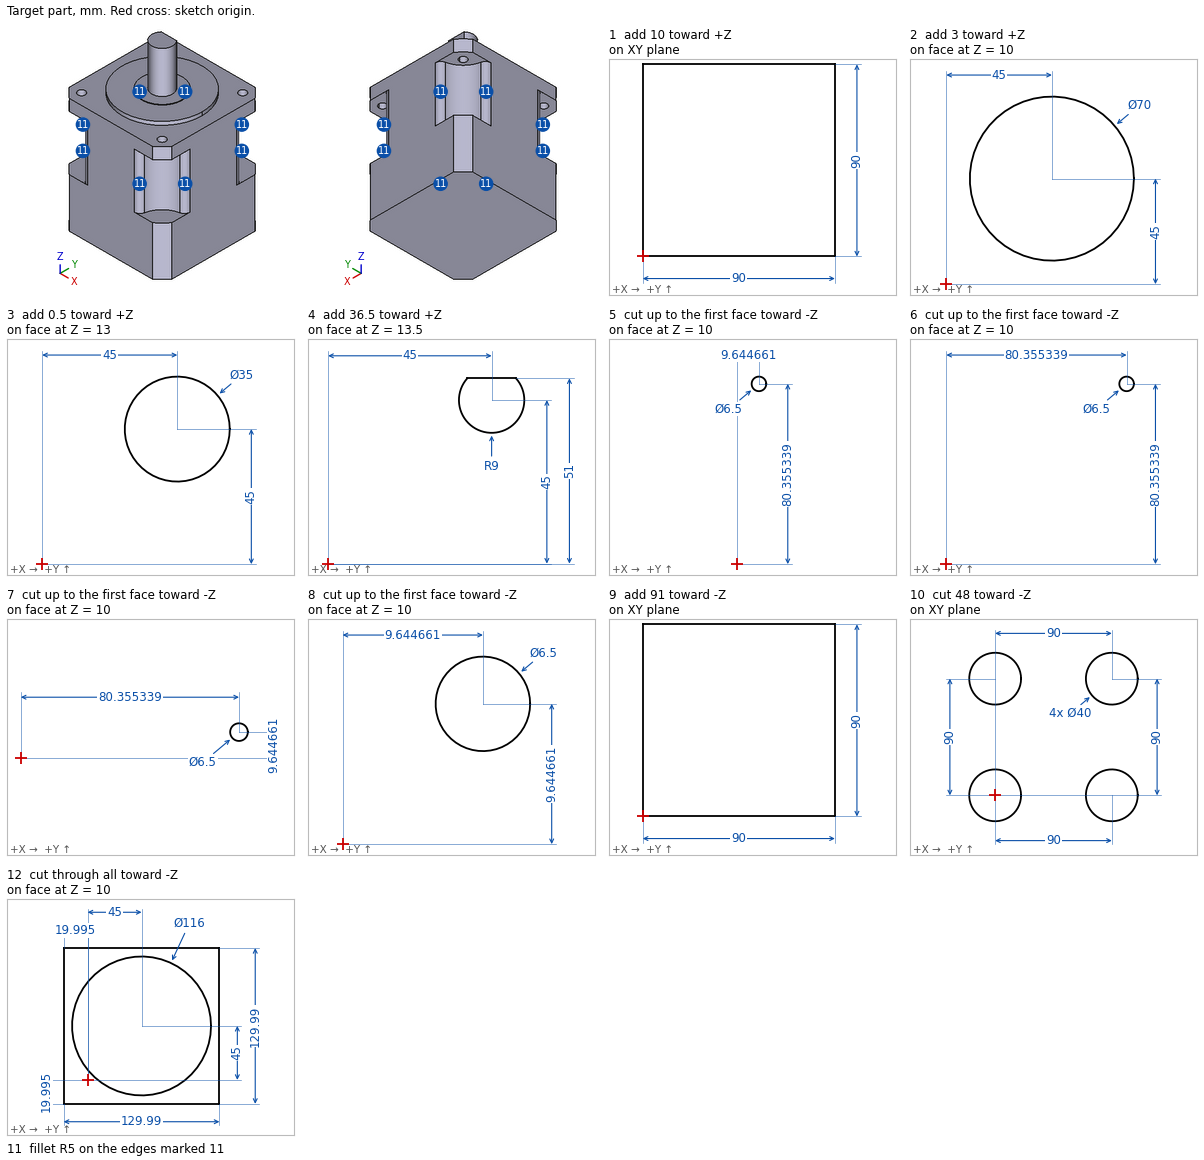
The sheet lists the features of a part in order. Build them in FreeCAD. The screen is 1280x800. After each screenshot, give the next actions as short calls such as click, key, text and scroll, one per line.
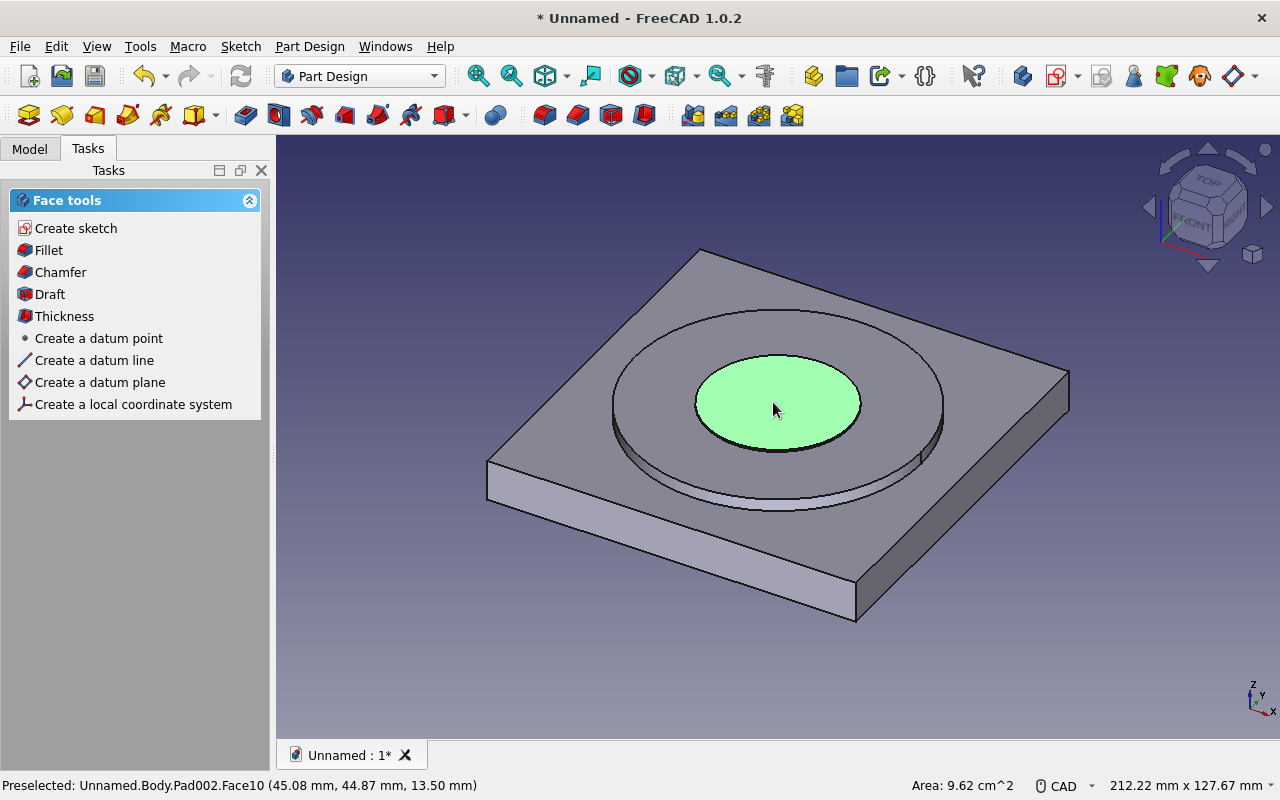
click(1056, 76)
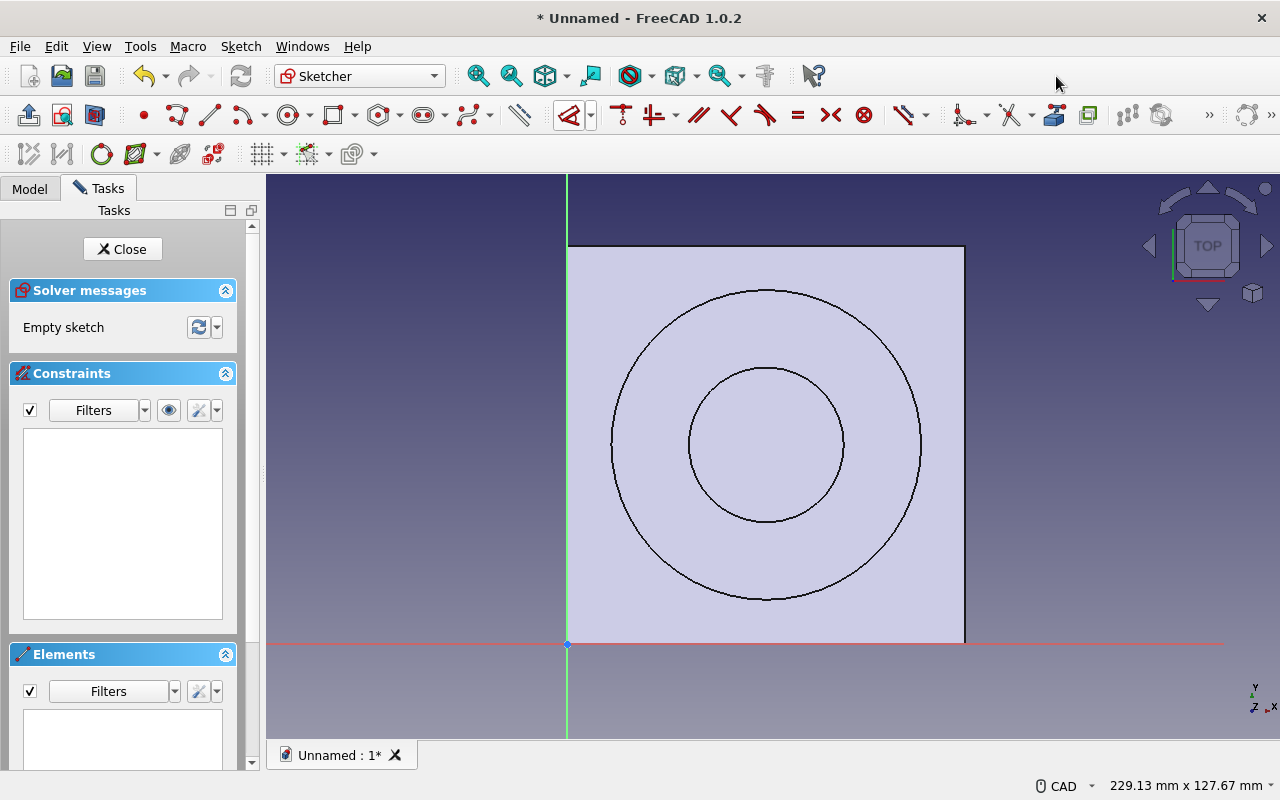
scroll(782, 450, up, 8)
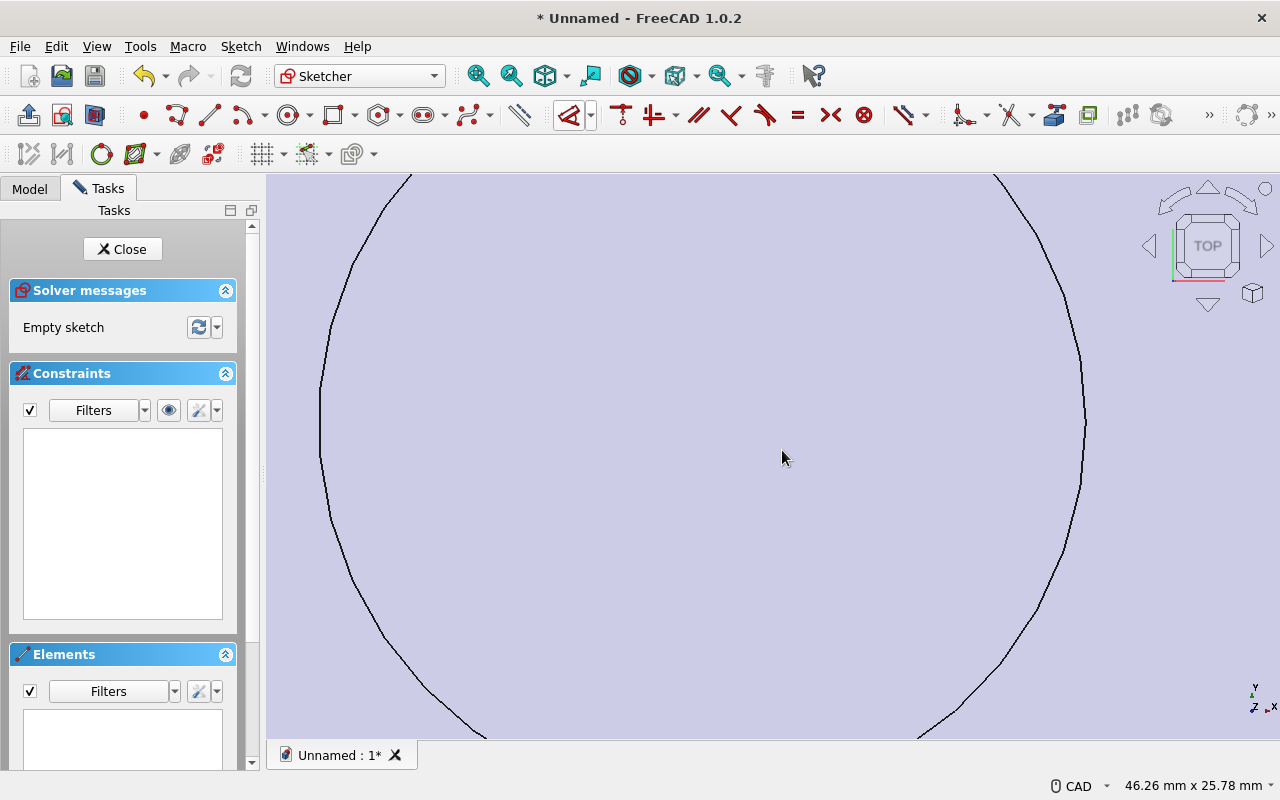
click(210, 116)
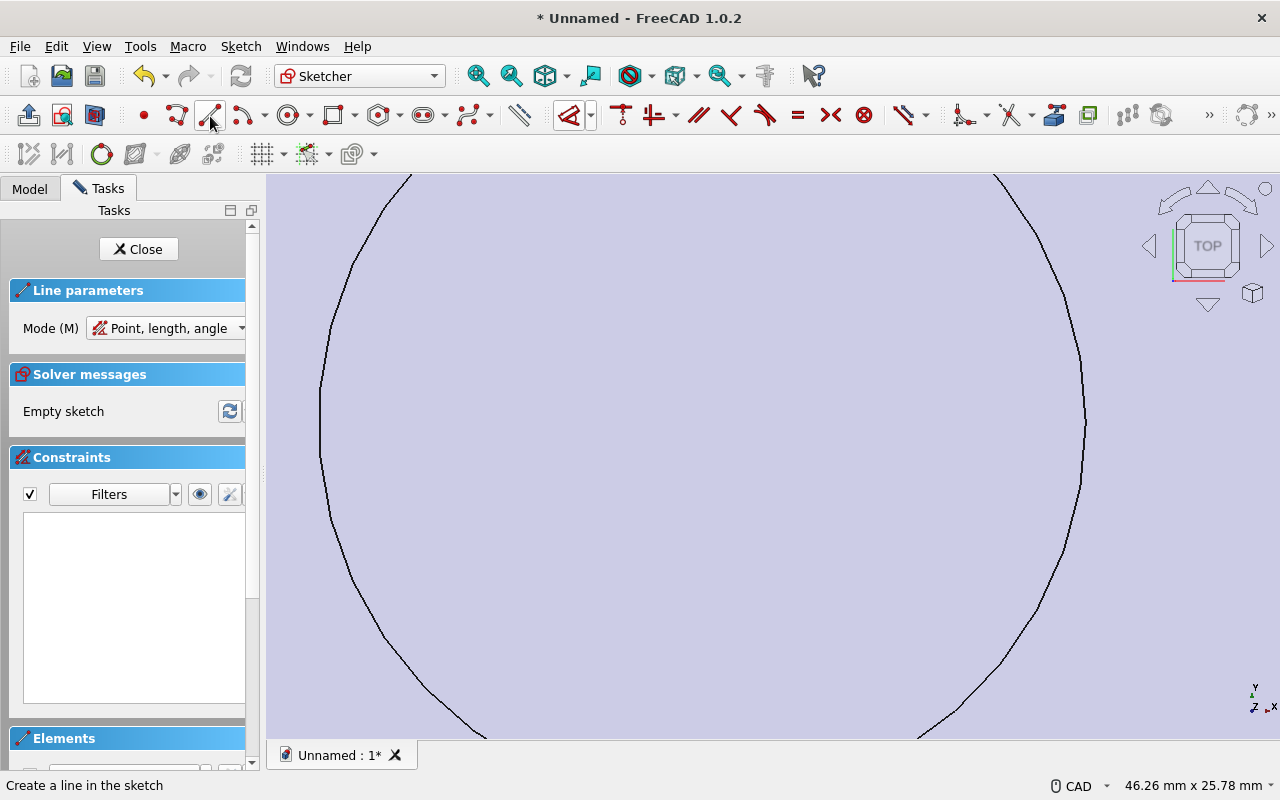
click(849, 291)
click(555, 291)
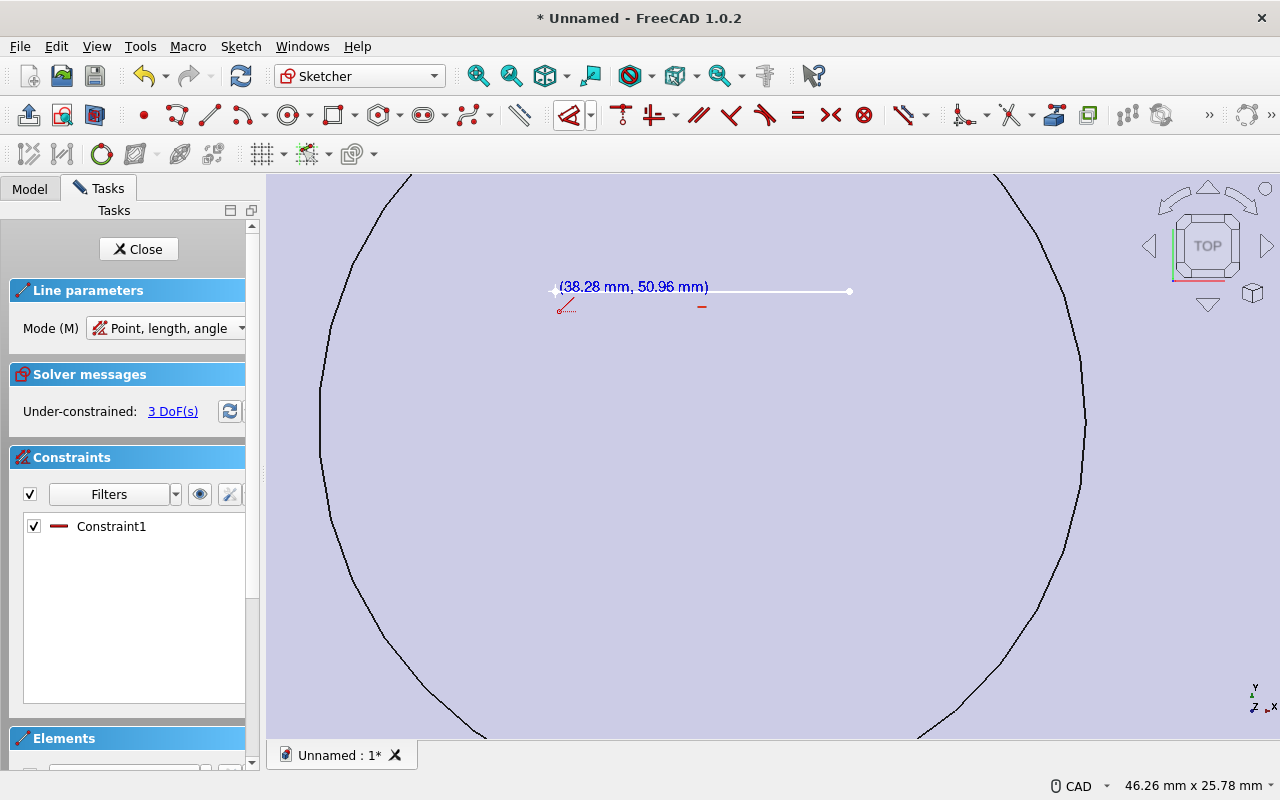
click(264, 116)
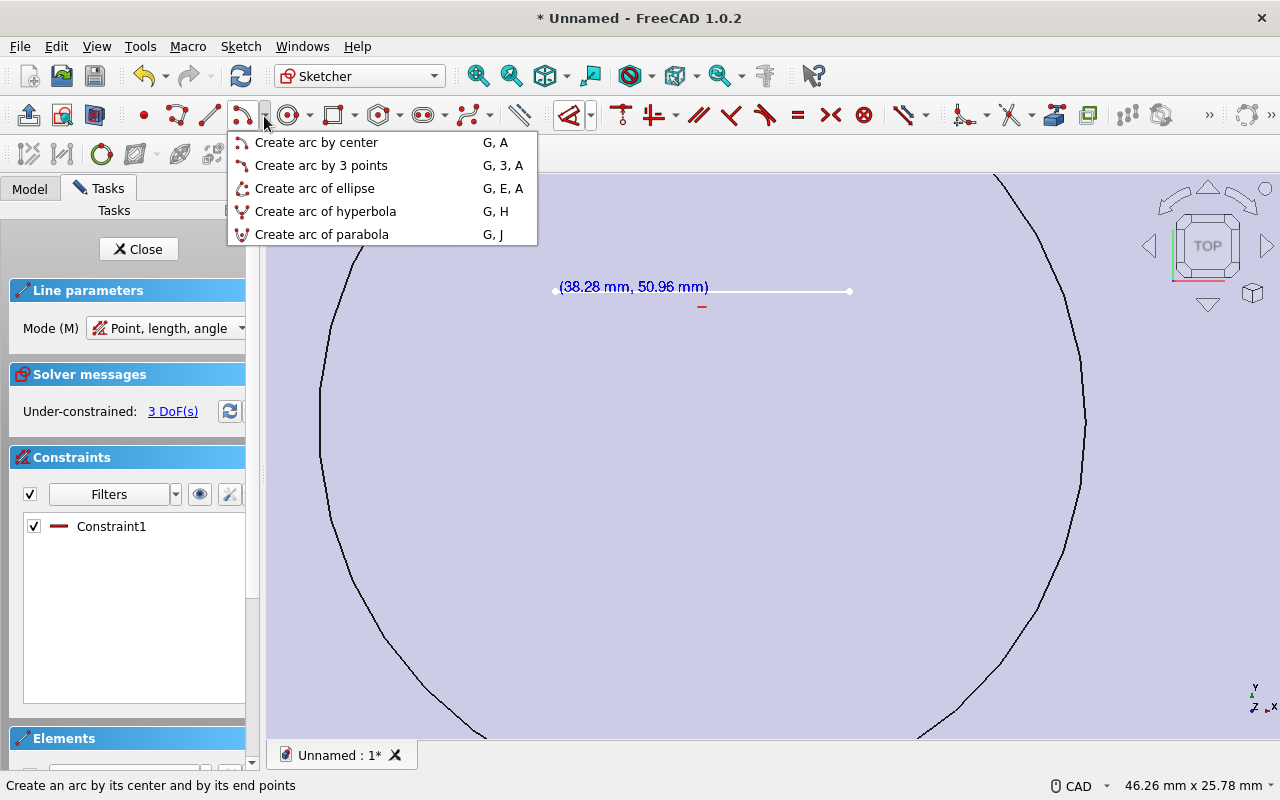
click(382, 166)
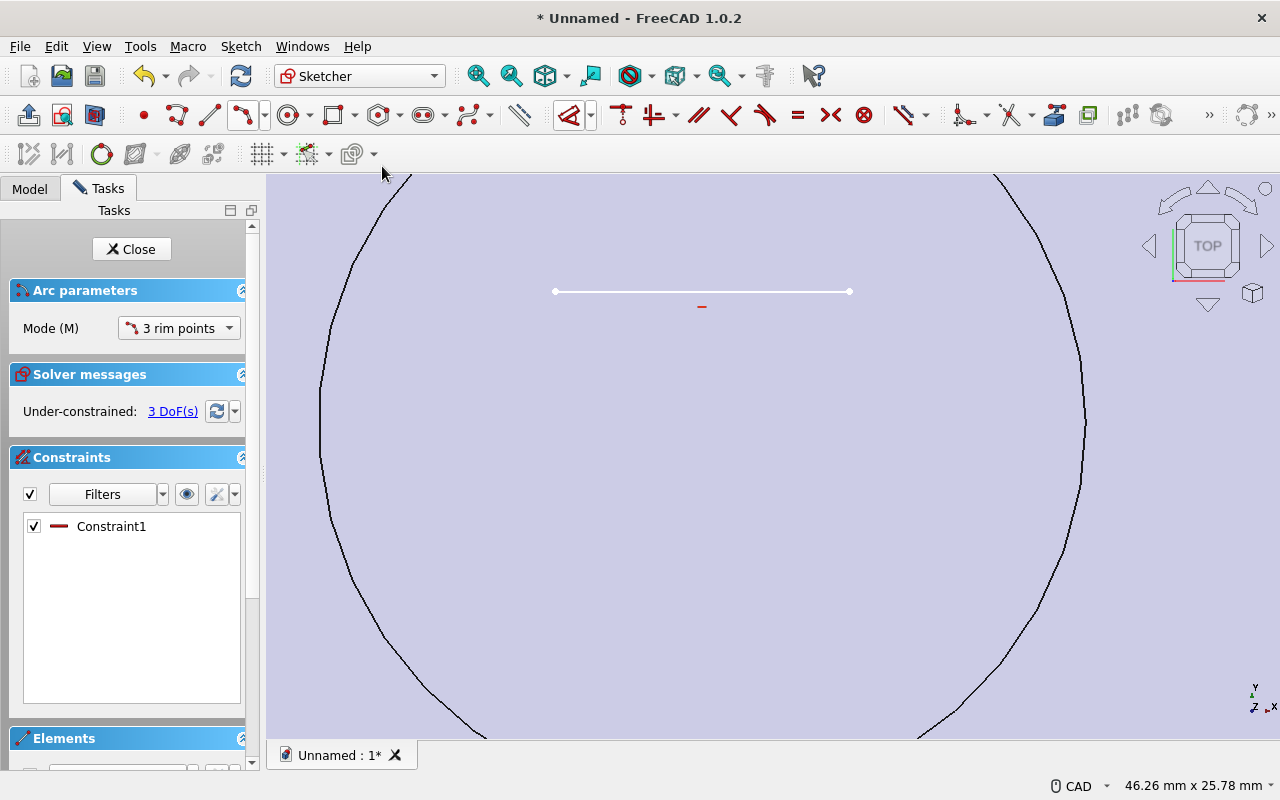
click(555, 292)
click(849, 292)
click(702, 620)
key(Escape)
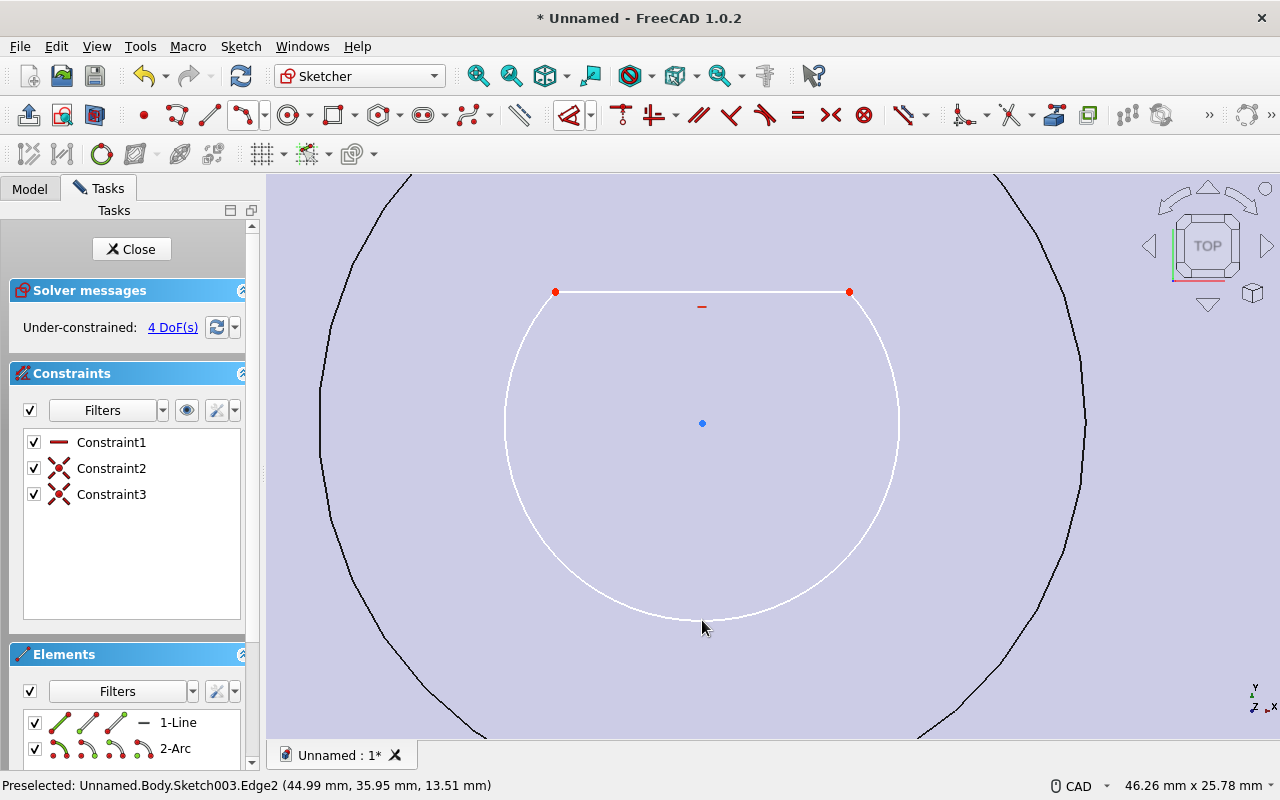
click(545, 543)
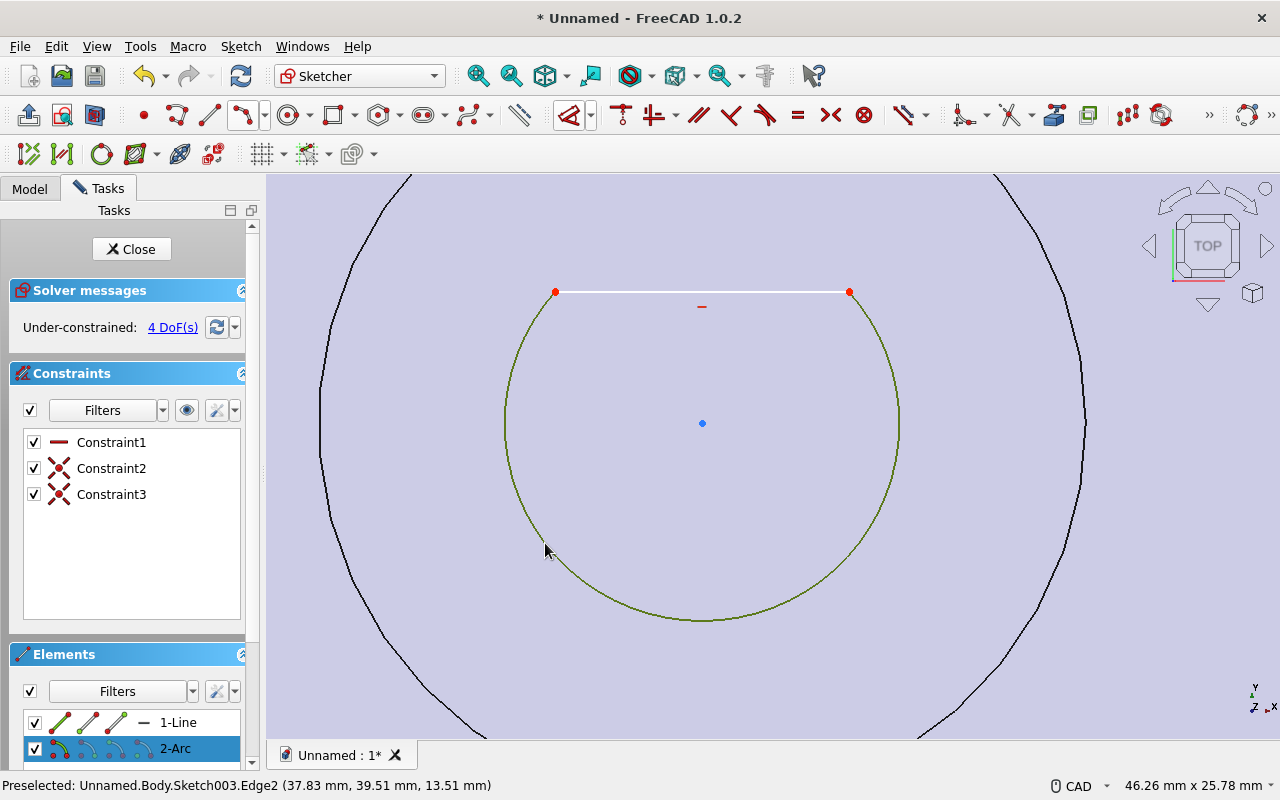
click(590, 116)